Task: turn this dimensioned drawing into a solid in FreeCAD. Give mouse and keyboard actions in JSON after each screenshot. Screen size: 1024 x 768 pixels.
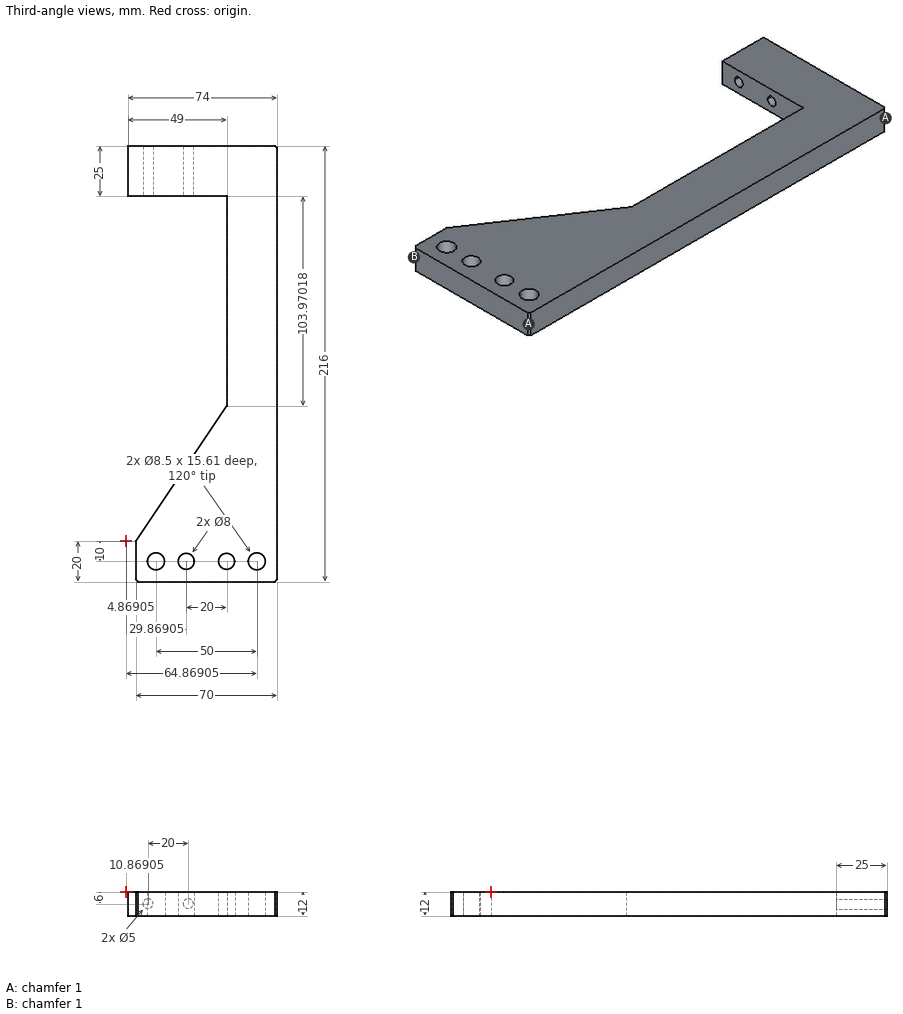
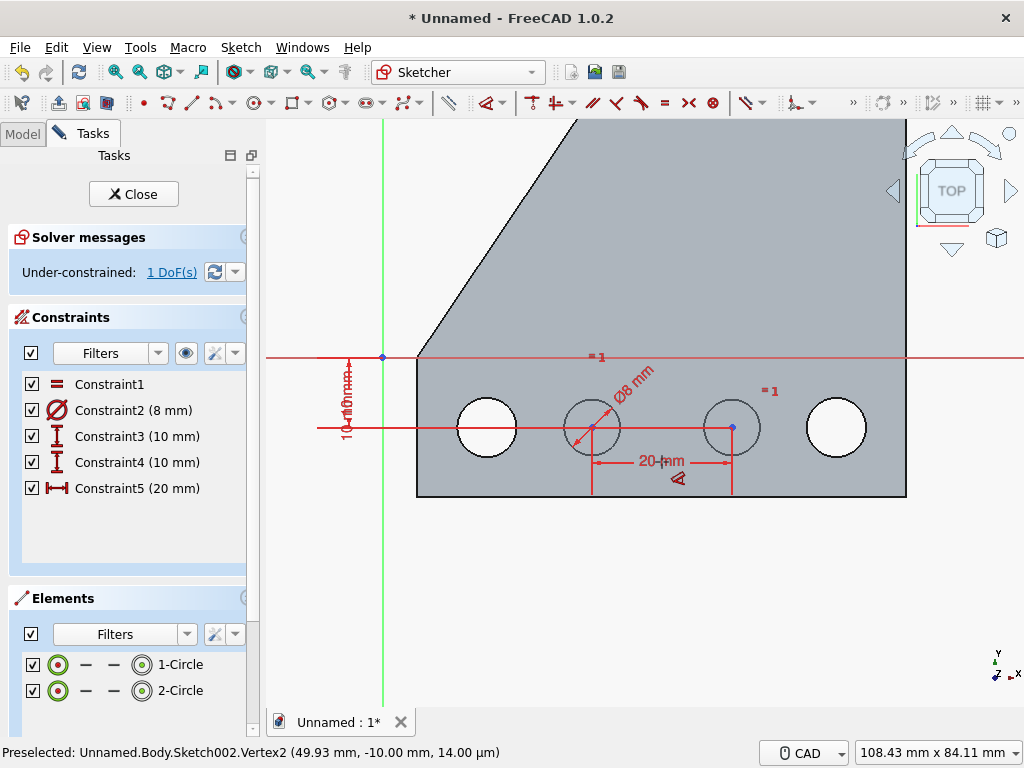
{"action": "left_click", "coordinate": [592, 428]}
{"action": "left_click", "coordinate": [488, 324]}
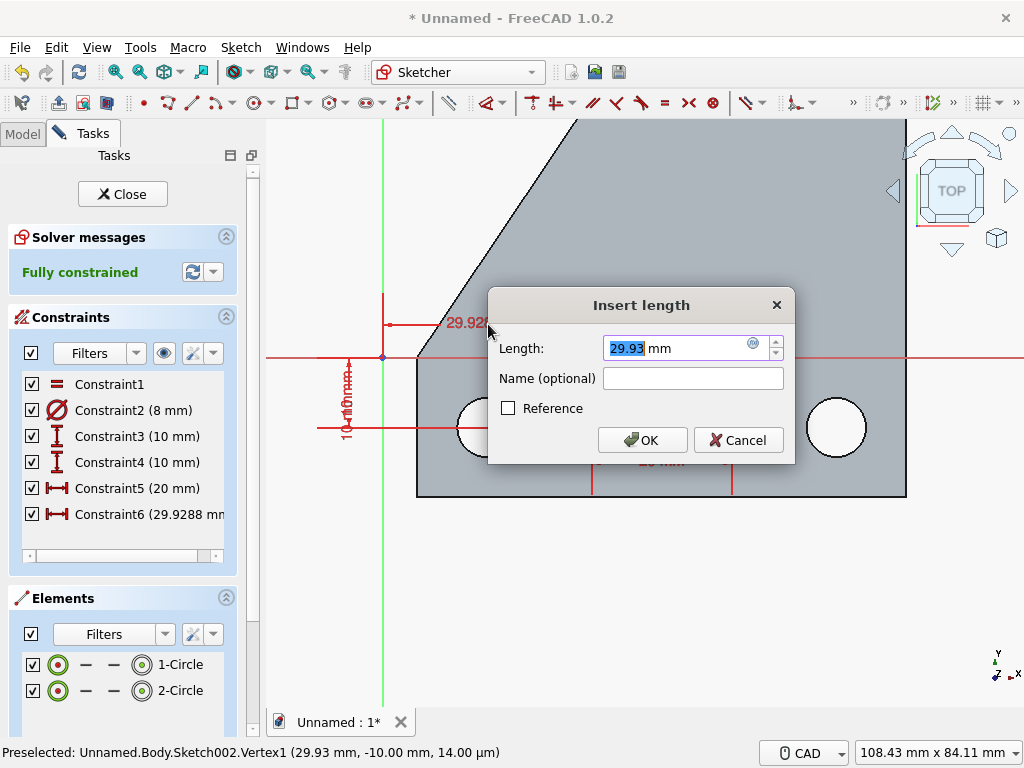
{"action": "type", "text": "29.86905"}
{"action": "key", "text": "Return"}
{"action": "key", "text": "Escape"}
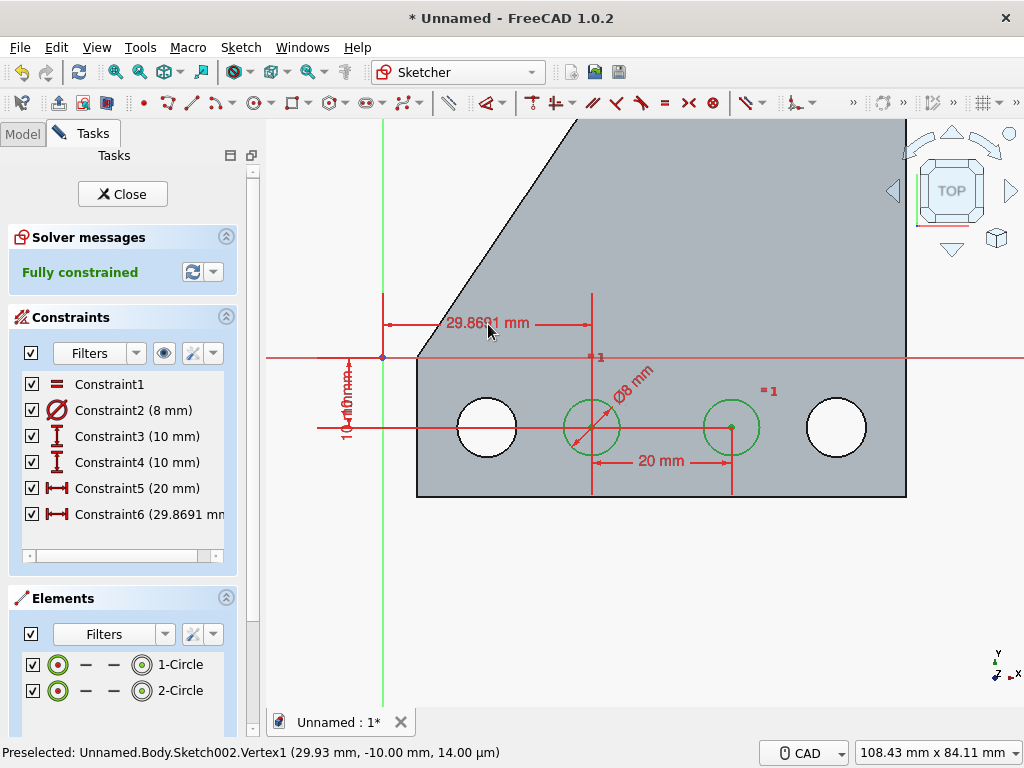
{"action": "left_click", "coordinate": [123, 194]}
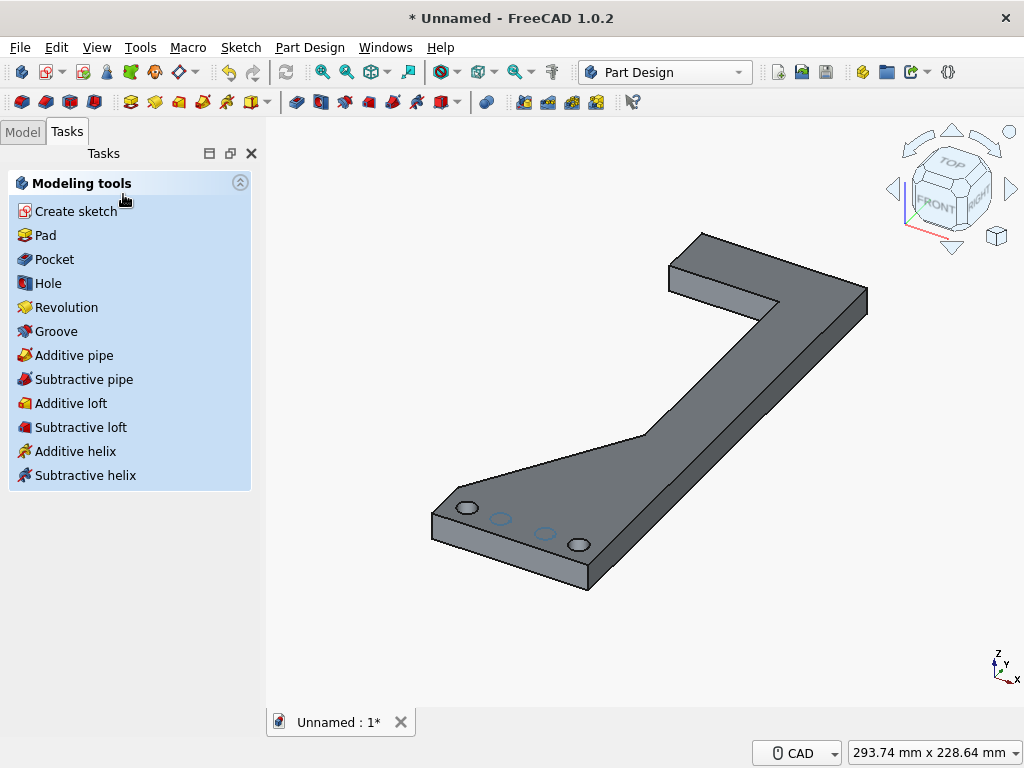
{"action": "left_click", "coordinate": [298, 102]}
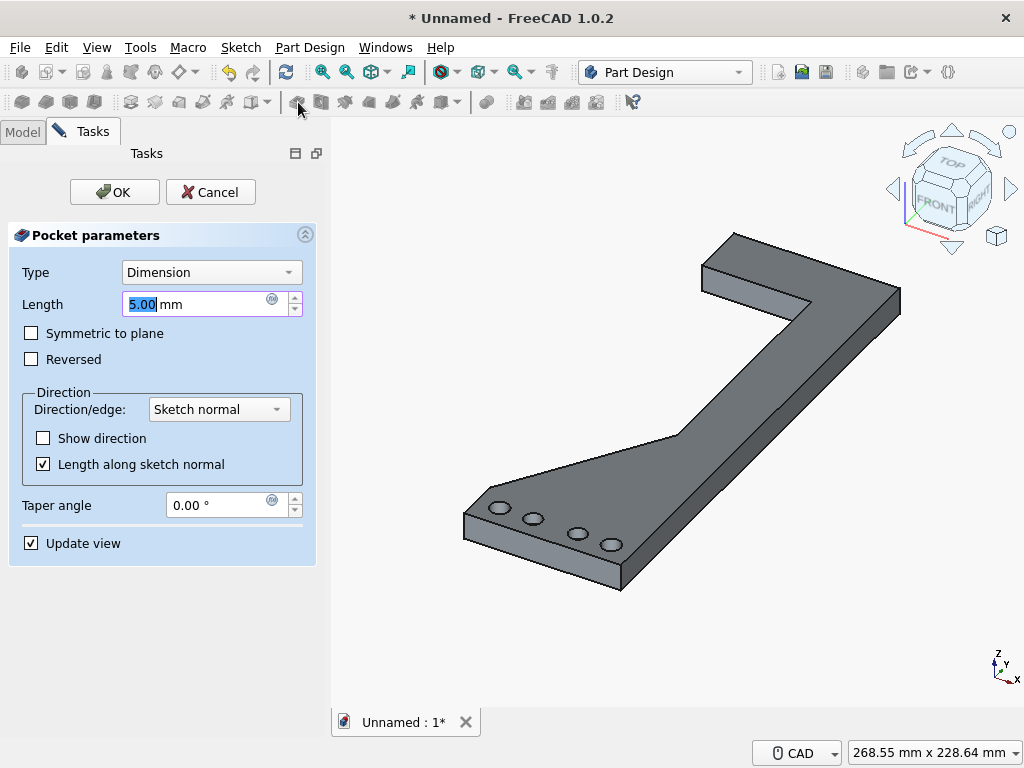
{"action": "type", "text": "12"}
{"action": "key", "text": "Tab"}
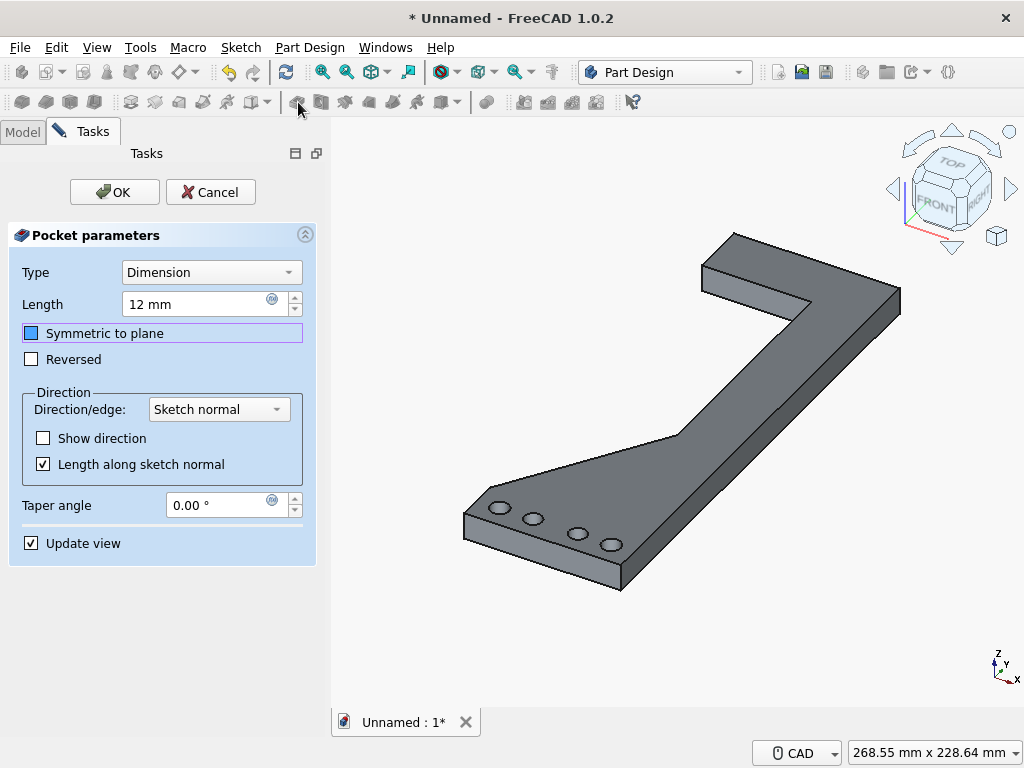
{"action": "left_click", "coordinate": [115, 192]}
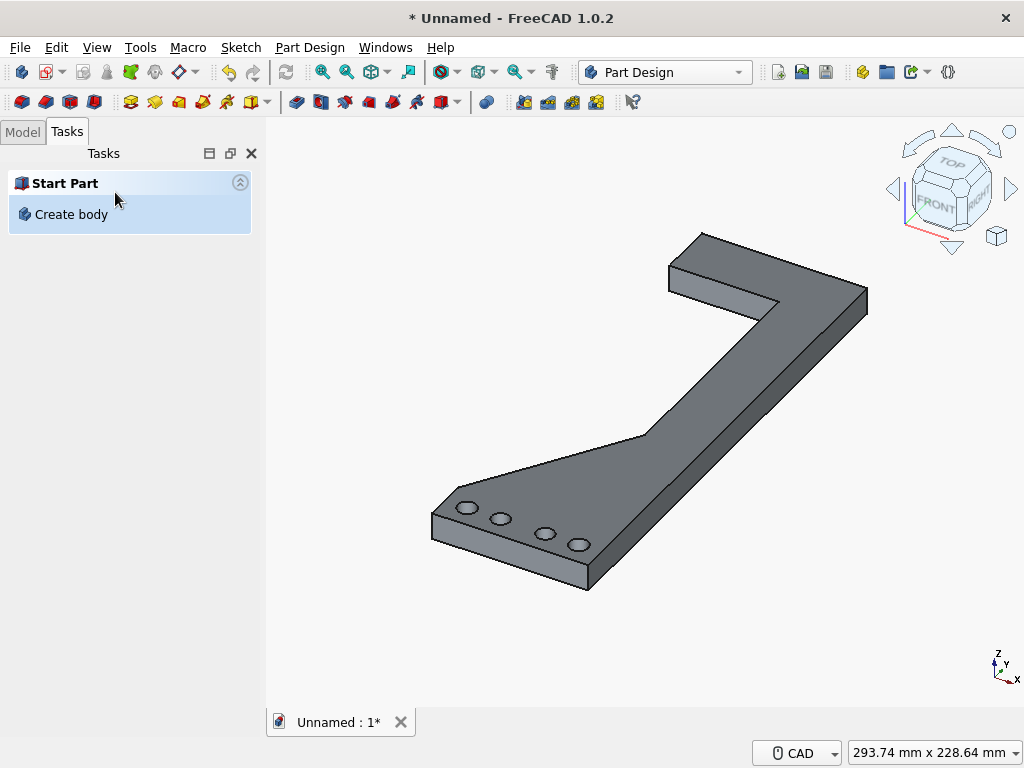
{"action": "key", "text": "4"}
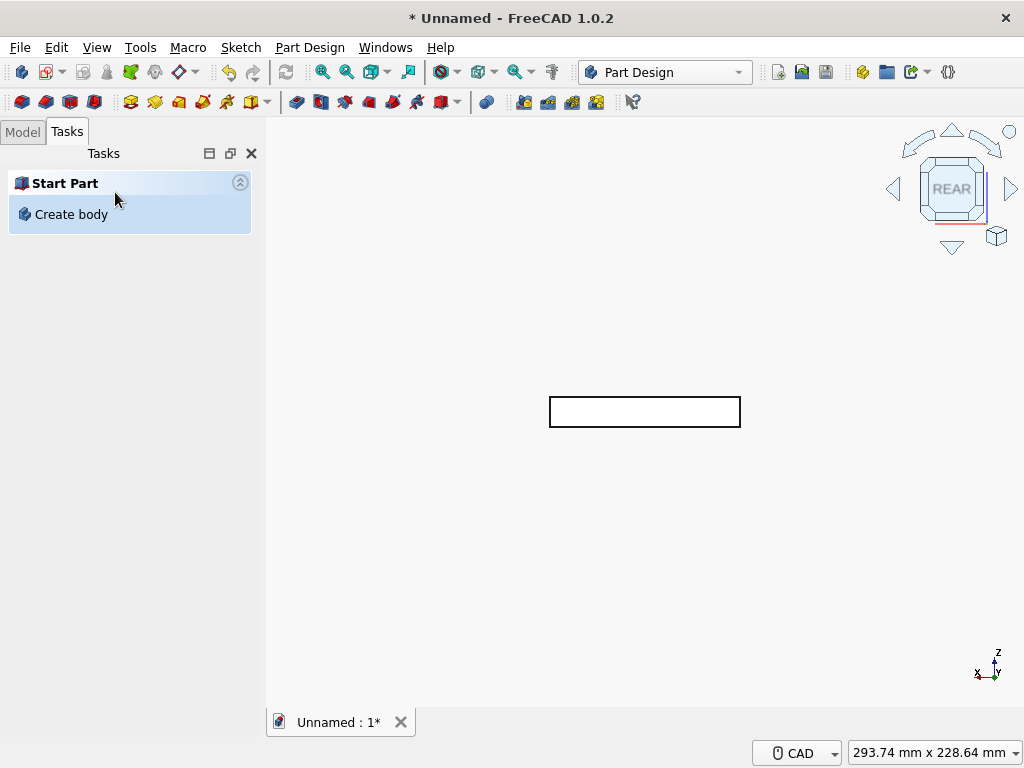
{"action": "key", "text": "v f"}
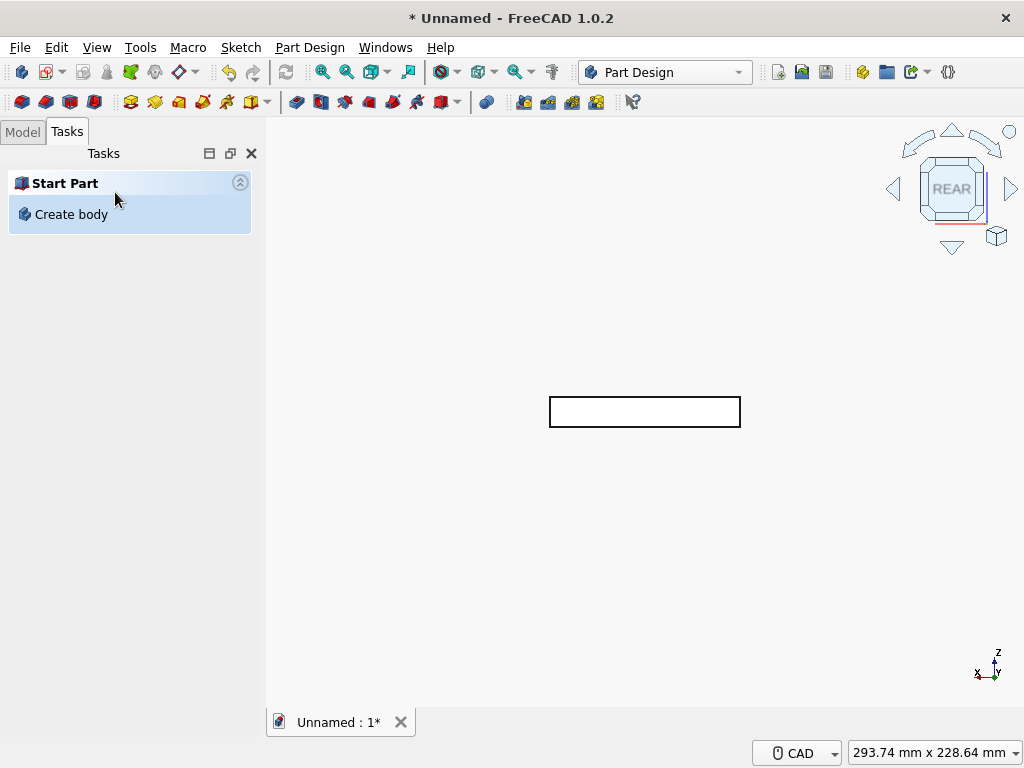
{"action": "left_click", "coordinate": [590, 411]}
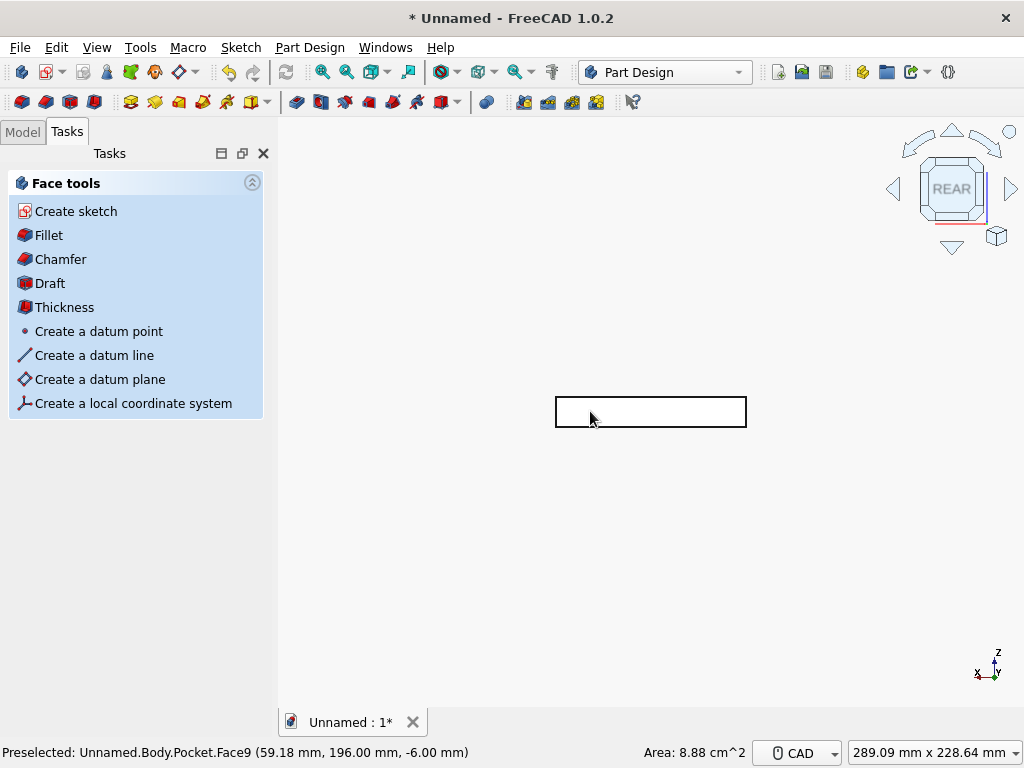
{"action": "left_click", "coordinate": [46, 72]}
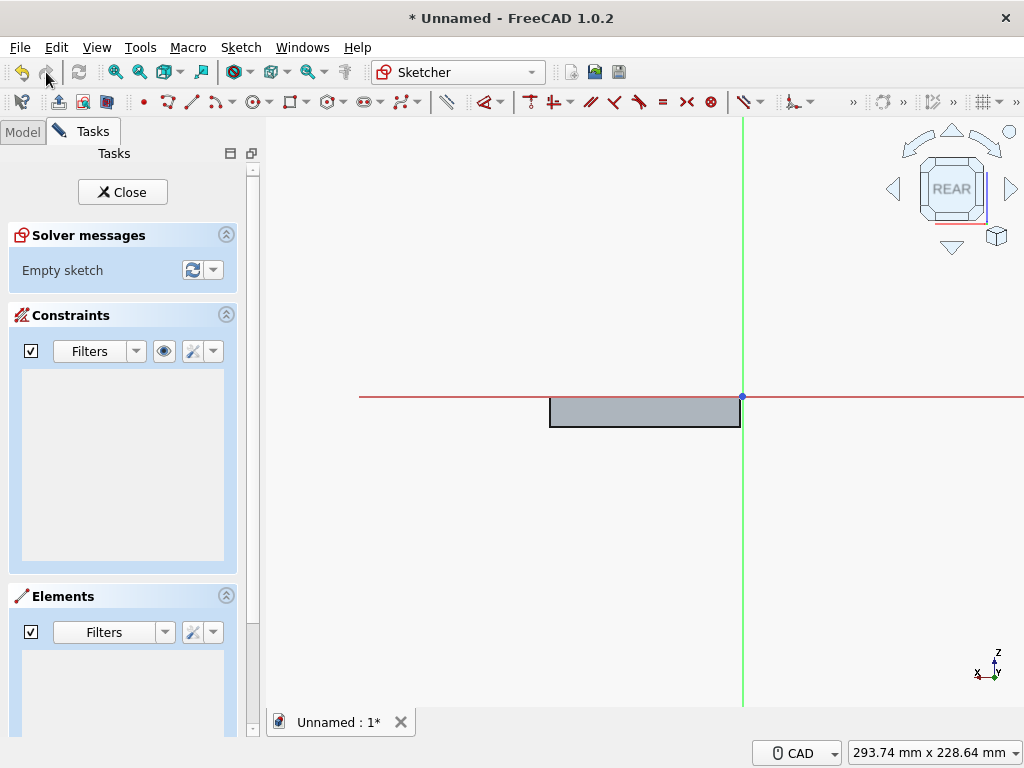
{"action": "scroll", "coordinate": [731, 406], "scroll_direction": "up", "scroll_amount": 8}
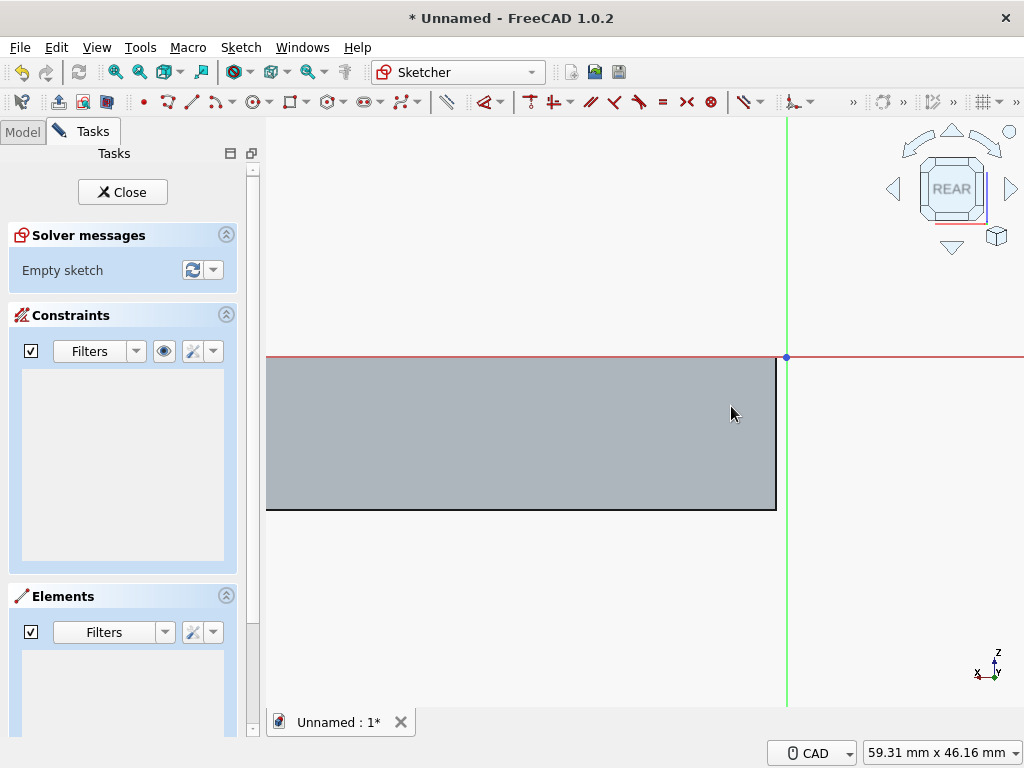
{"action": "key", "text": "g c"}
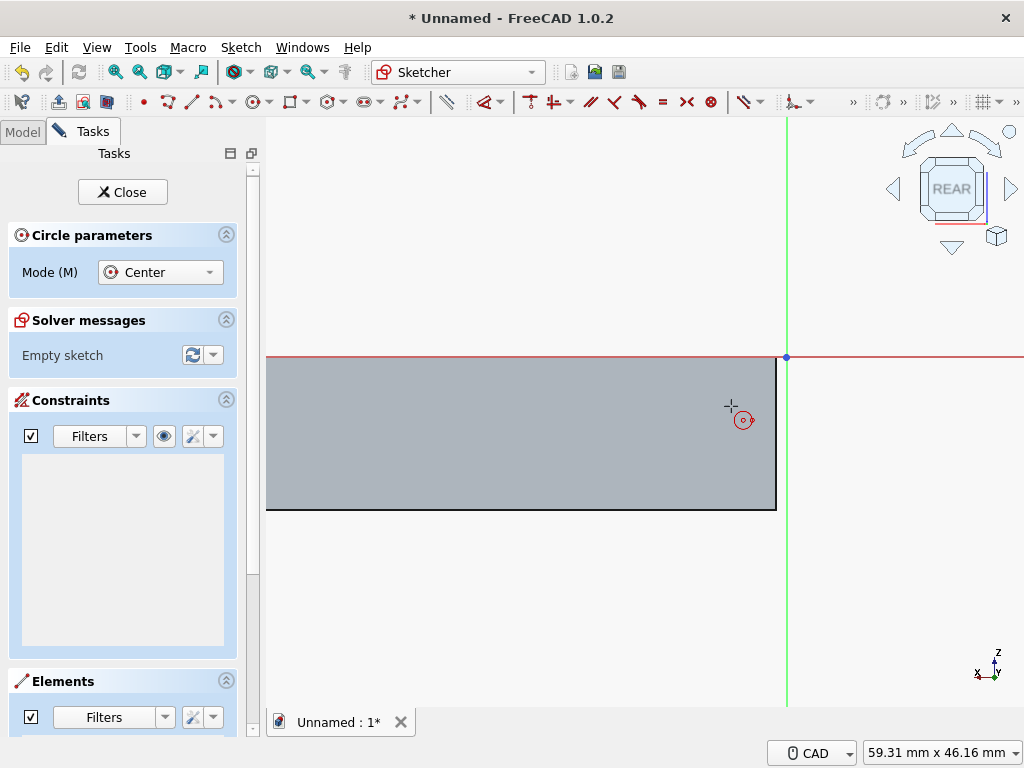
{"action": "left_click", "coordinate": [648, 434]}
{"action": "left_click", "coordinate": [670, 411]}